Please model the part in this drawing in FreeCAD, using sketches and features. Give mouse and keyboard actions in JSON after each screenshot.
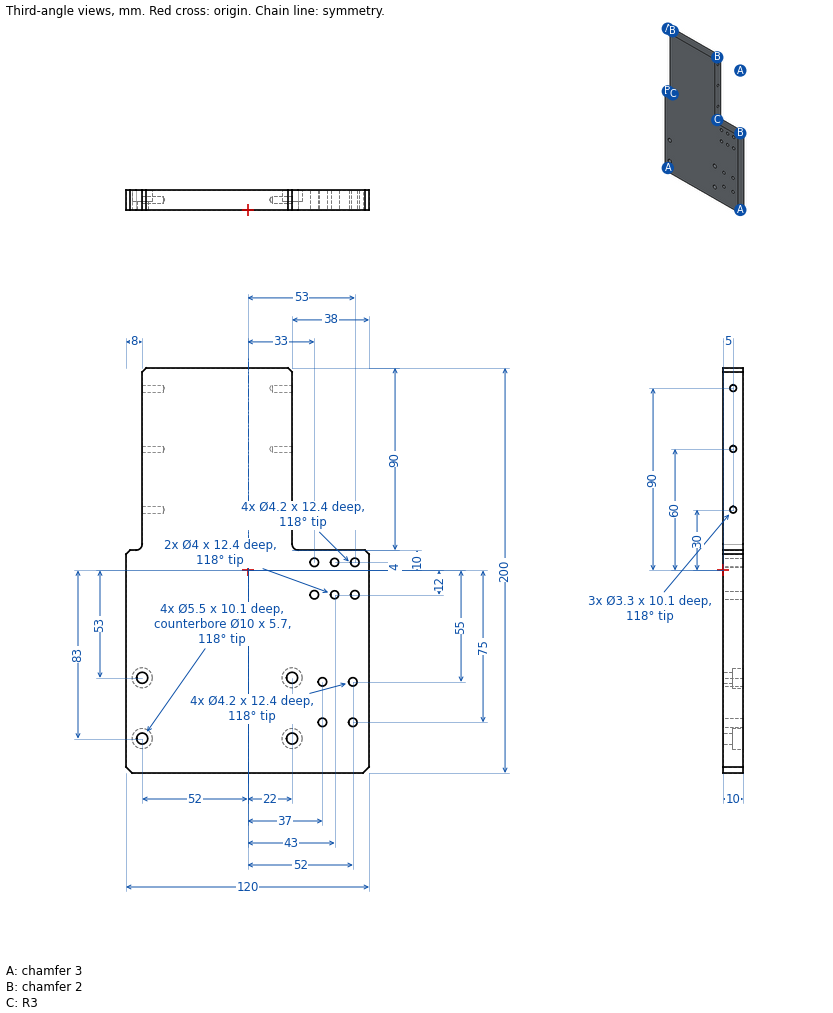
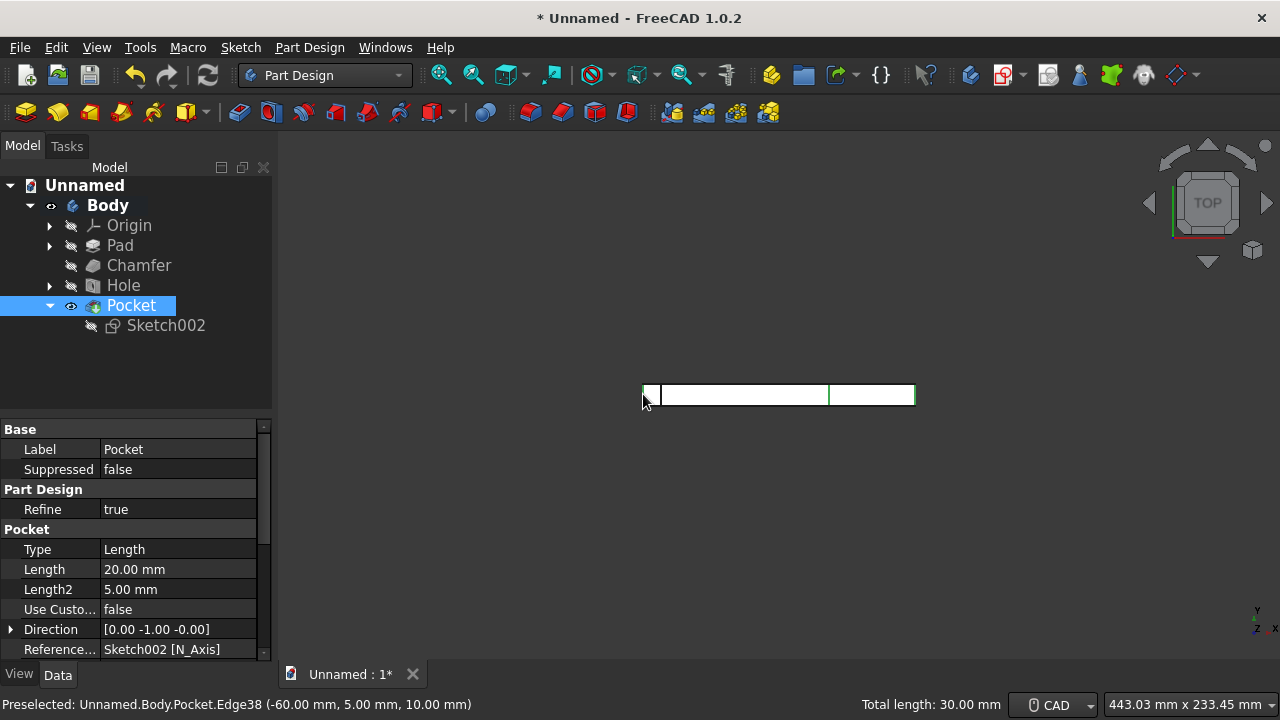
{"action": "left_click", "coordinate": [661, 394], "text": "ctrl"}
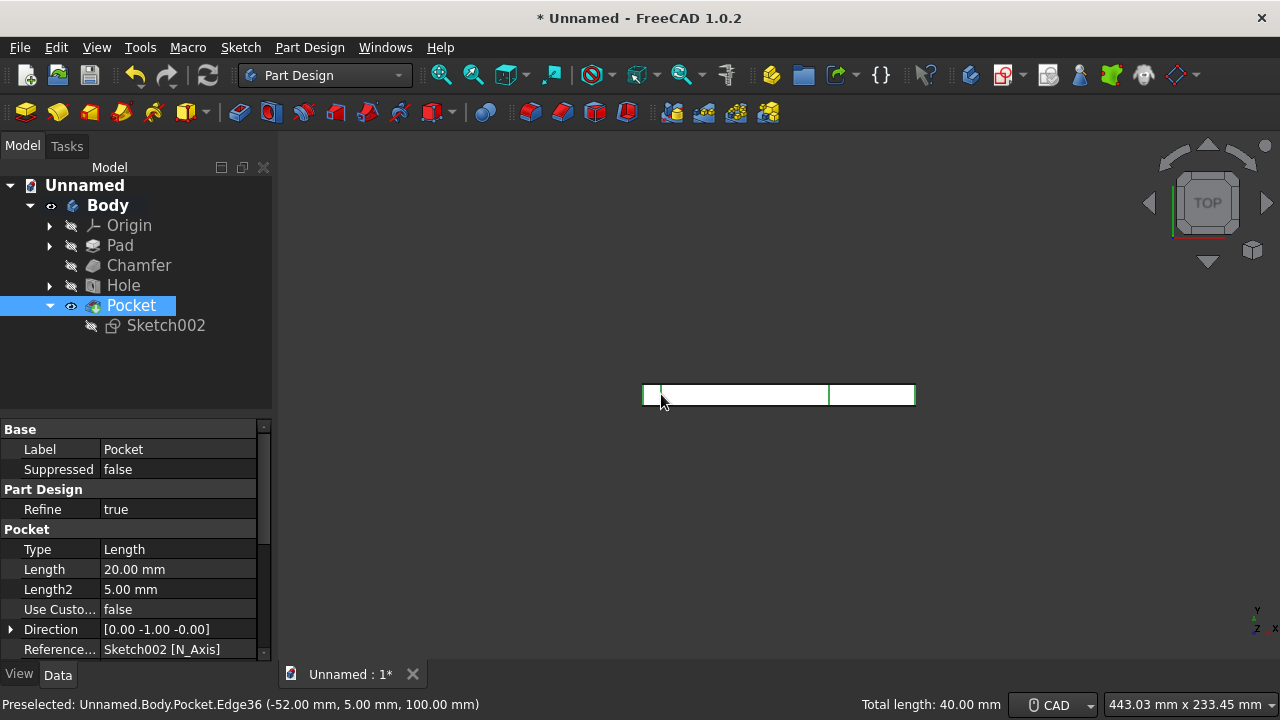
{"action": "left_click", "coordinate": [564, 112]}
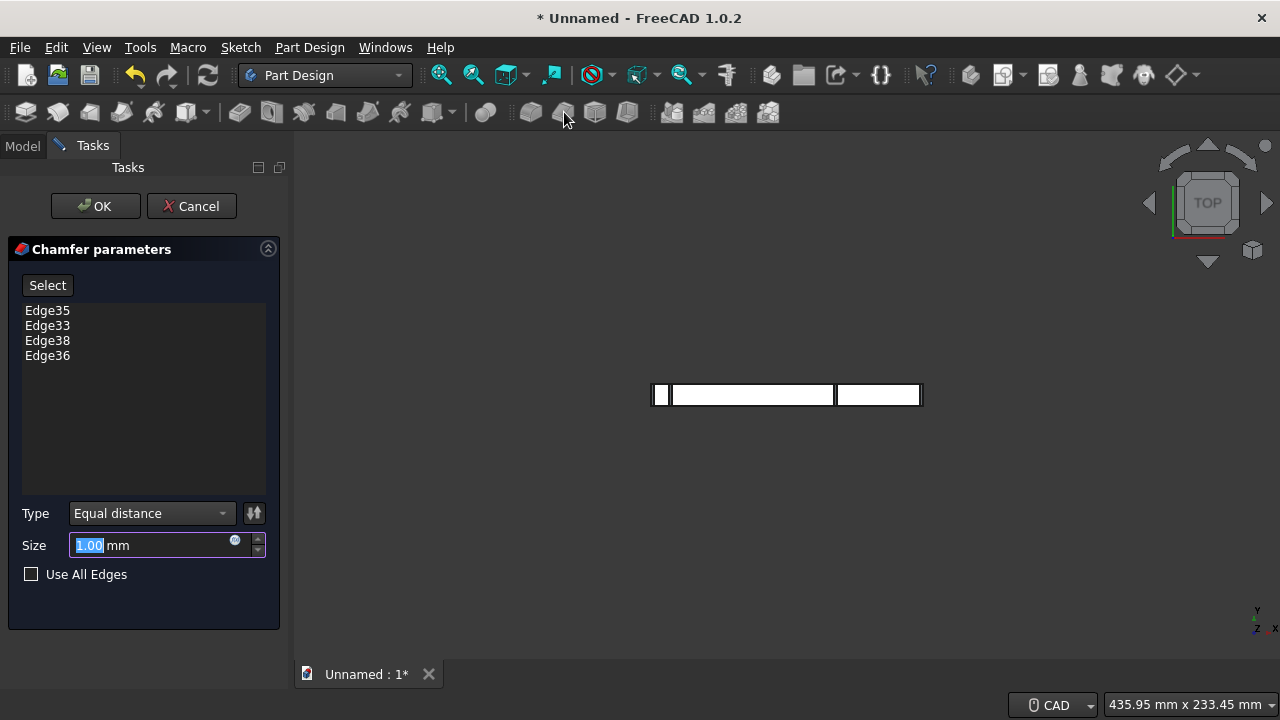
{"action": "type", "text": "2"}
{"action": "key", "text": "Tab"}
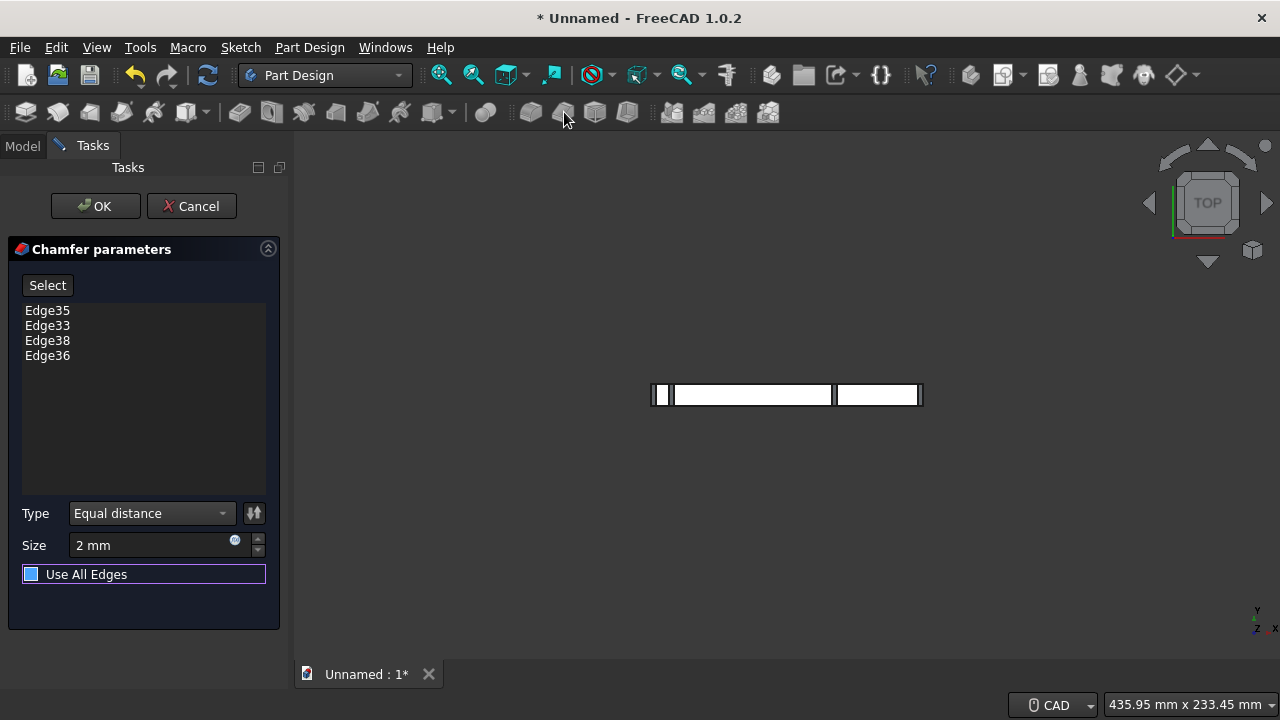
{"action": "left_click", "coordinate": [96, 206]}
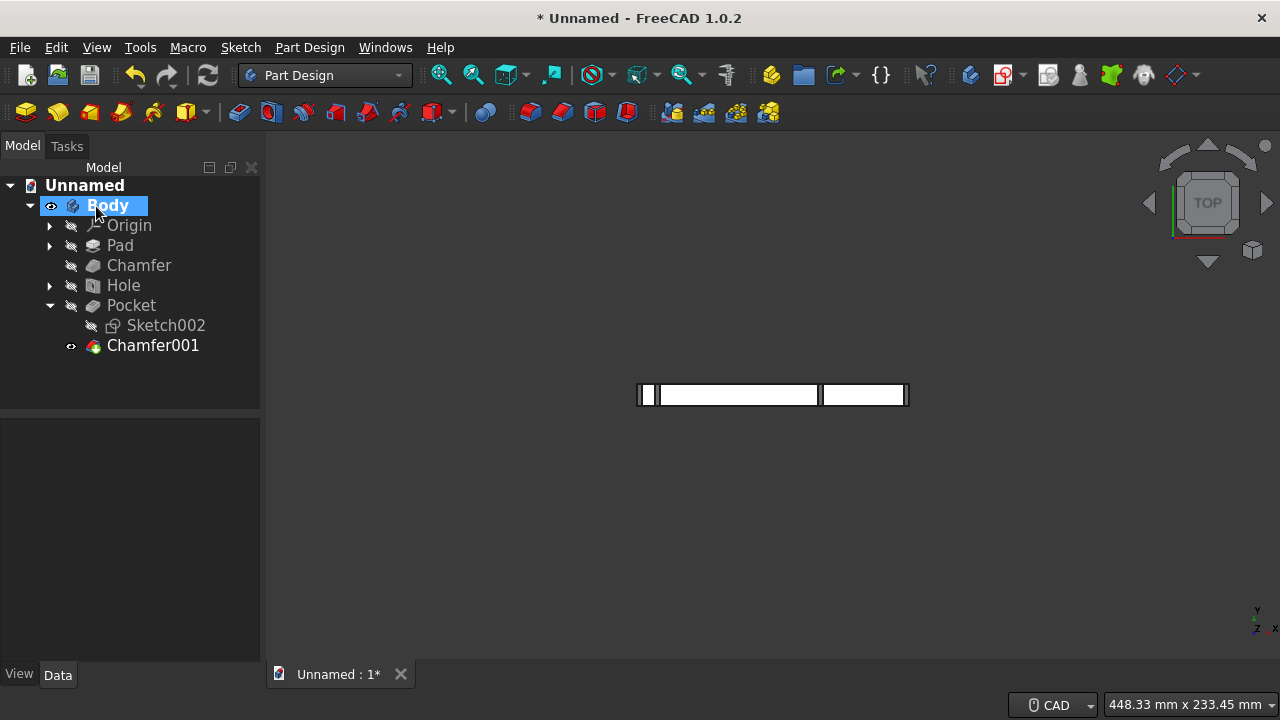
{"action": "left_click", "coordinate": [442, 76]}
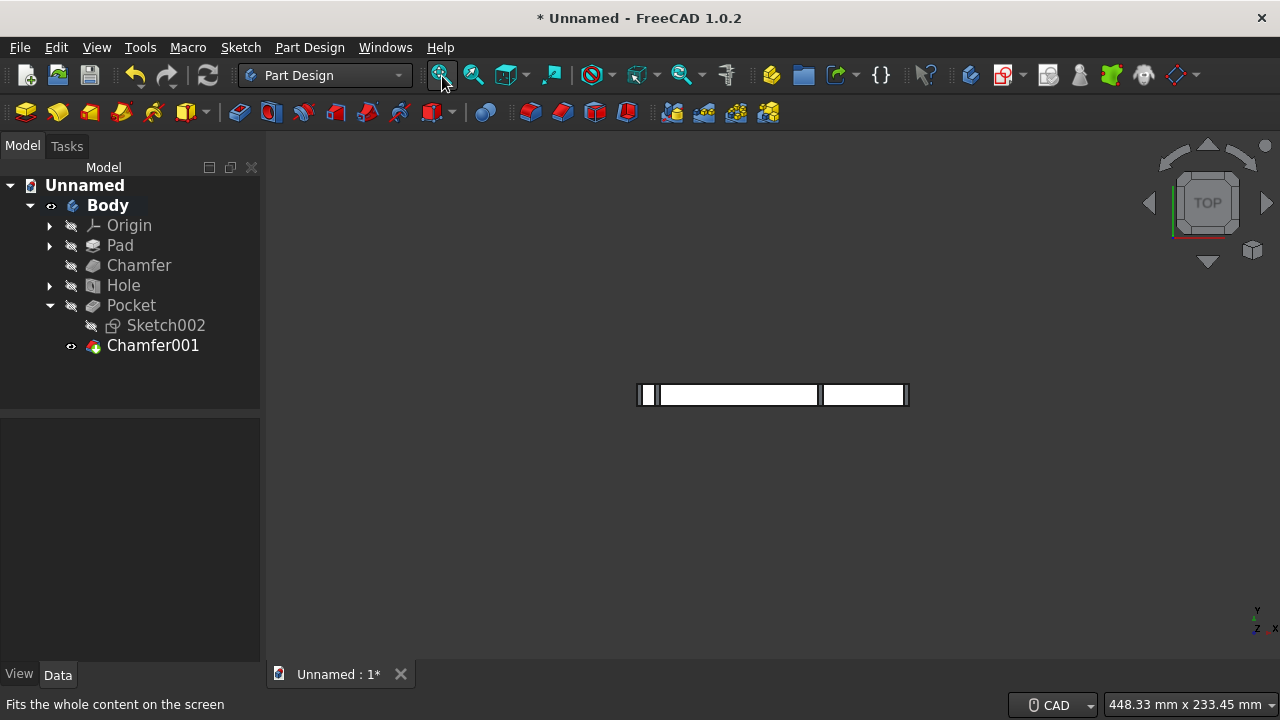
{"action": "key", "text": "0"}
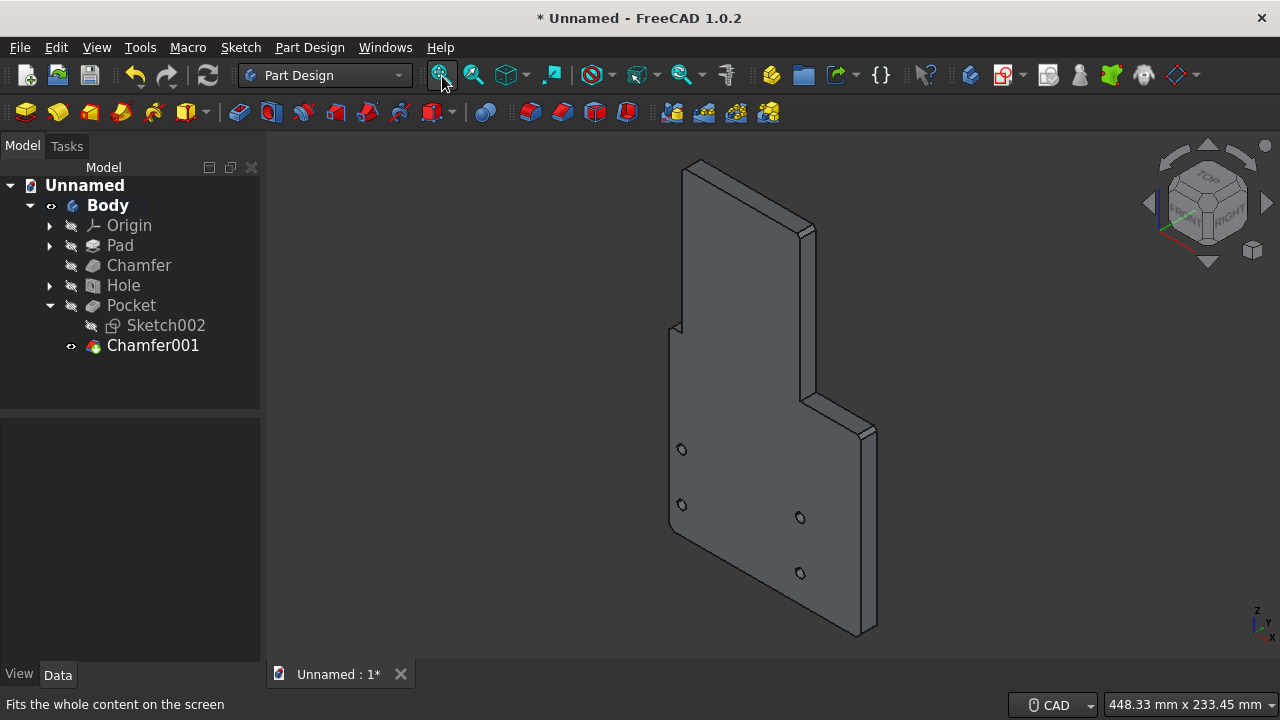
{"action": "key", "text": "2"}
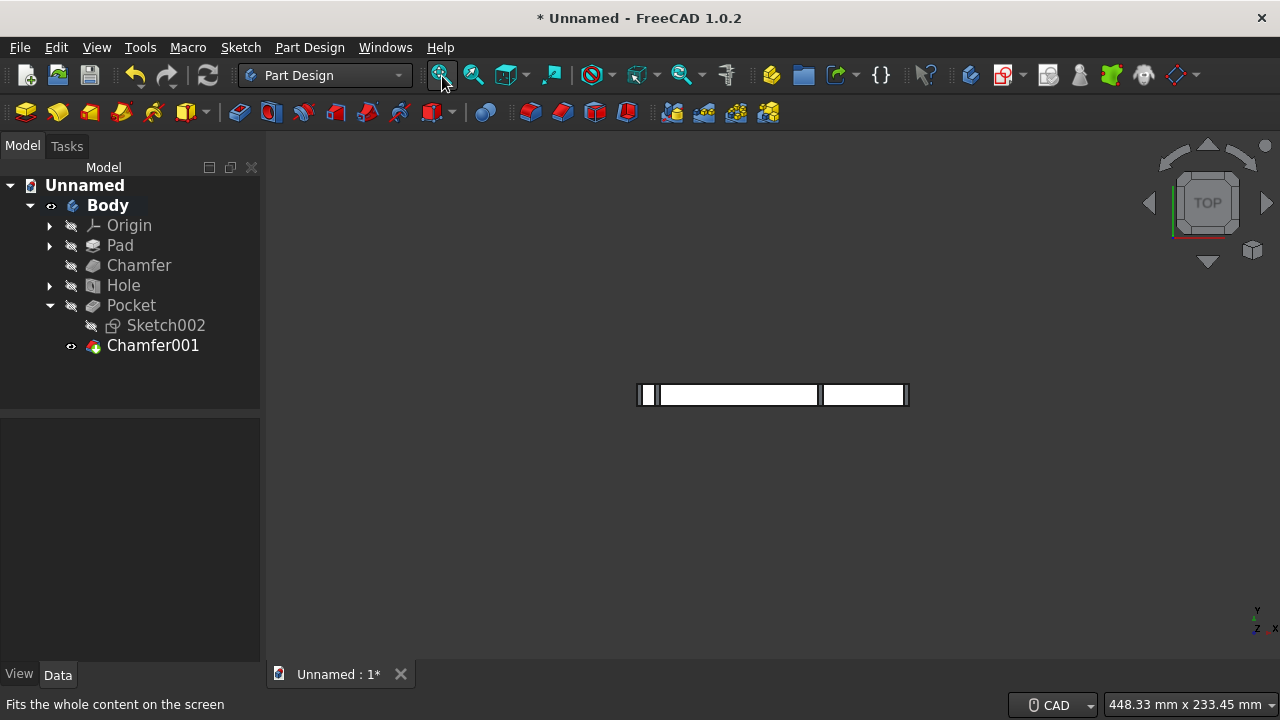
{"action": "left_click", "coordinate": [442, 76]}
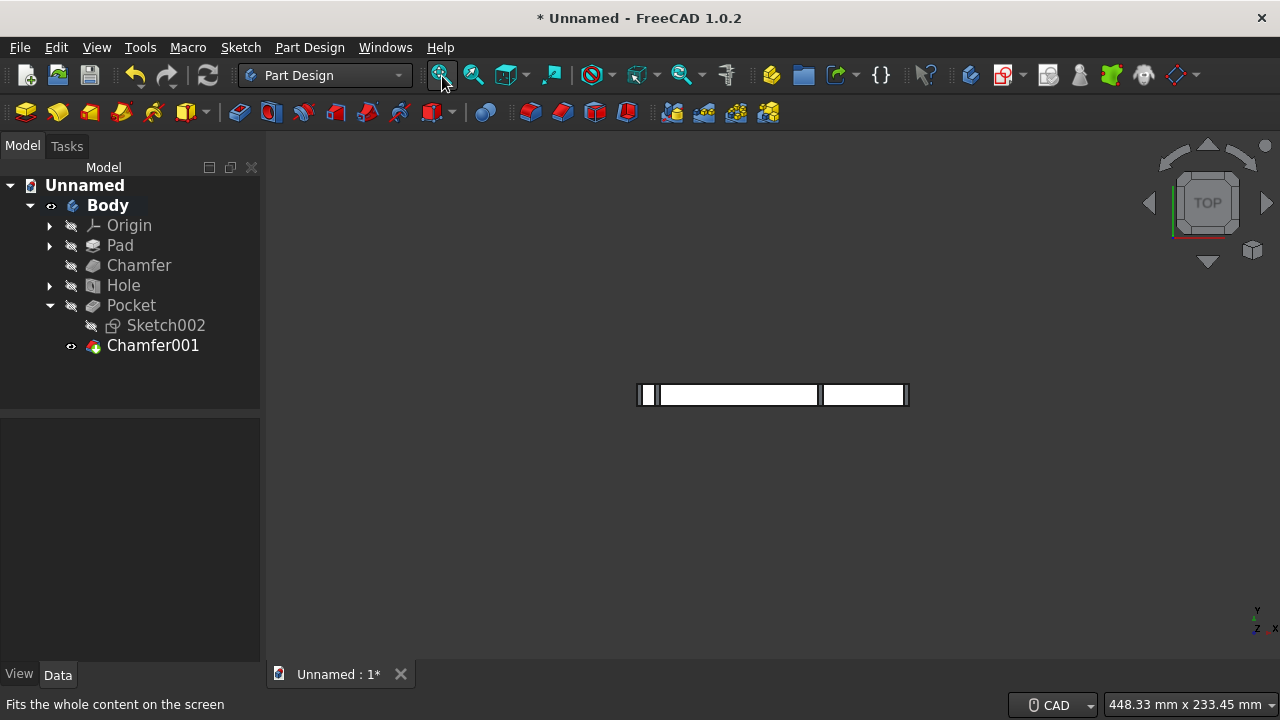
{"action": "key", "text": "1"}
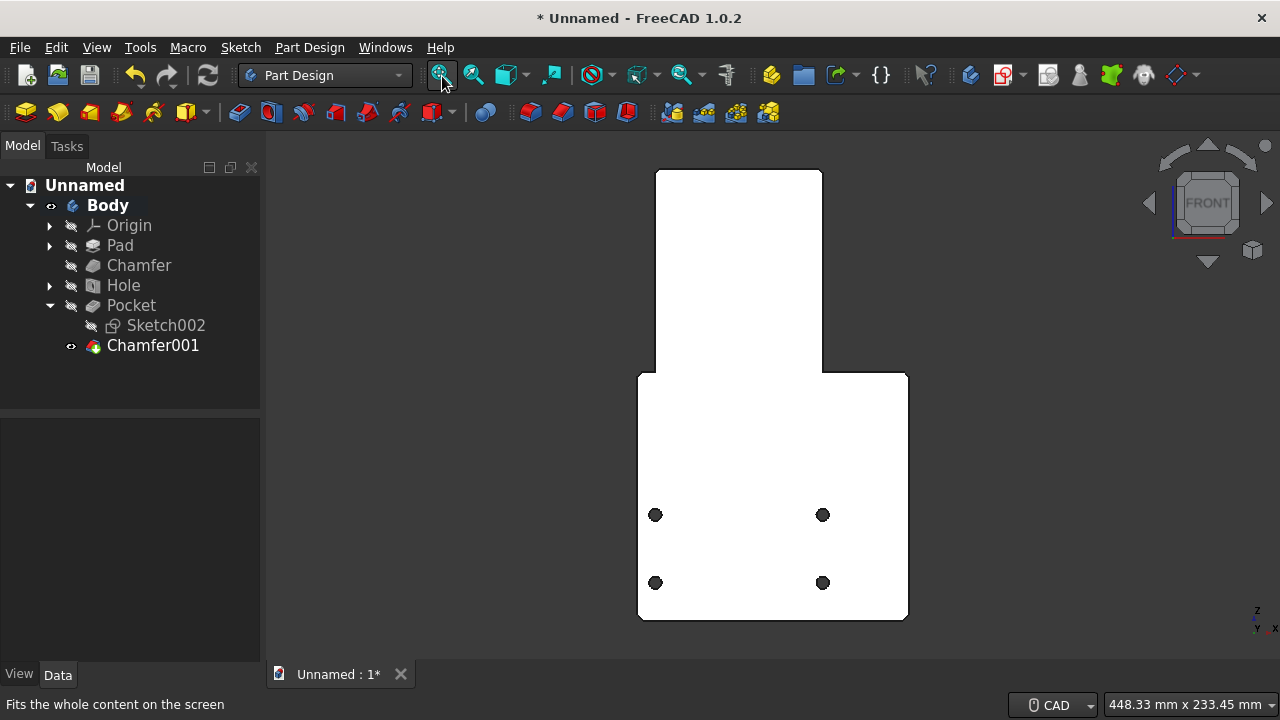
{"action": "key", "text": "3"}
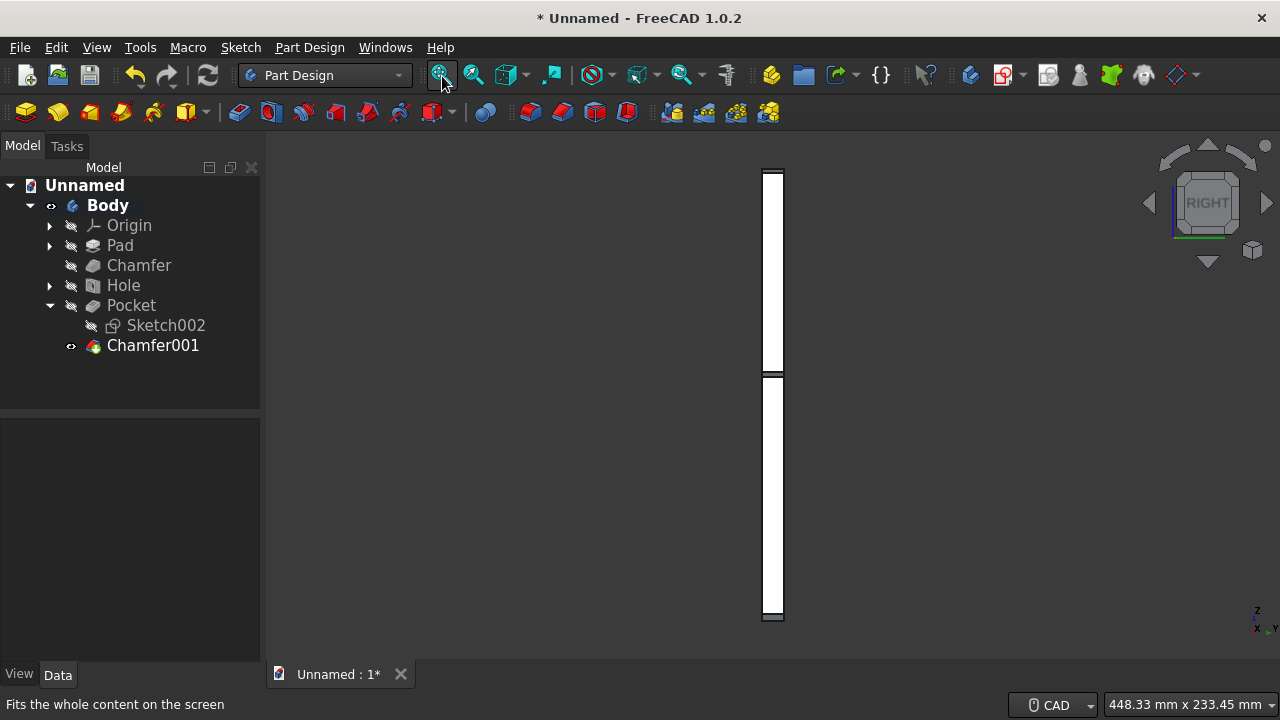
{"action": "key", "text": "5"}